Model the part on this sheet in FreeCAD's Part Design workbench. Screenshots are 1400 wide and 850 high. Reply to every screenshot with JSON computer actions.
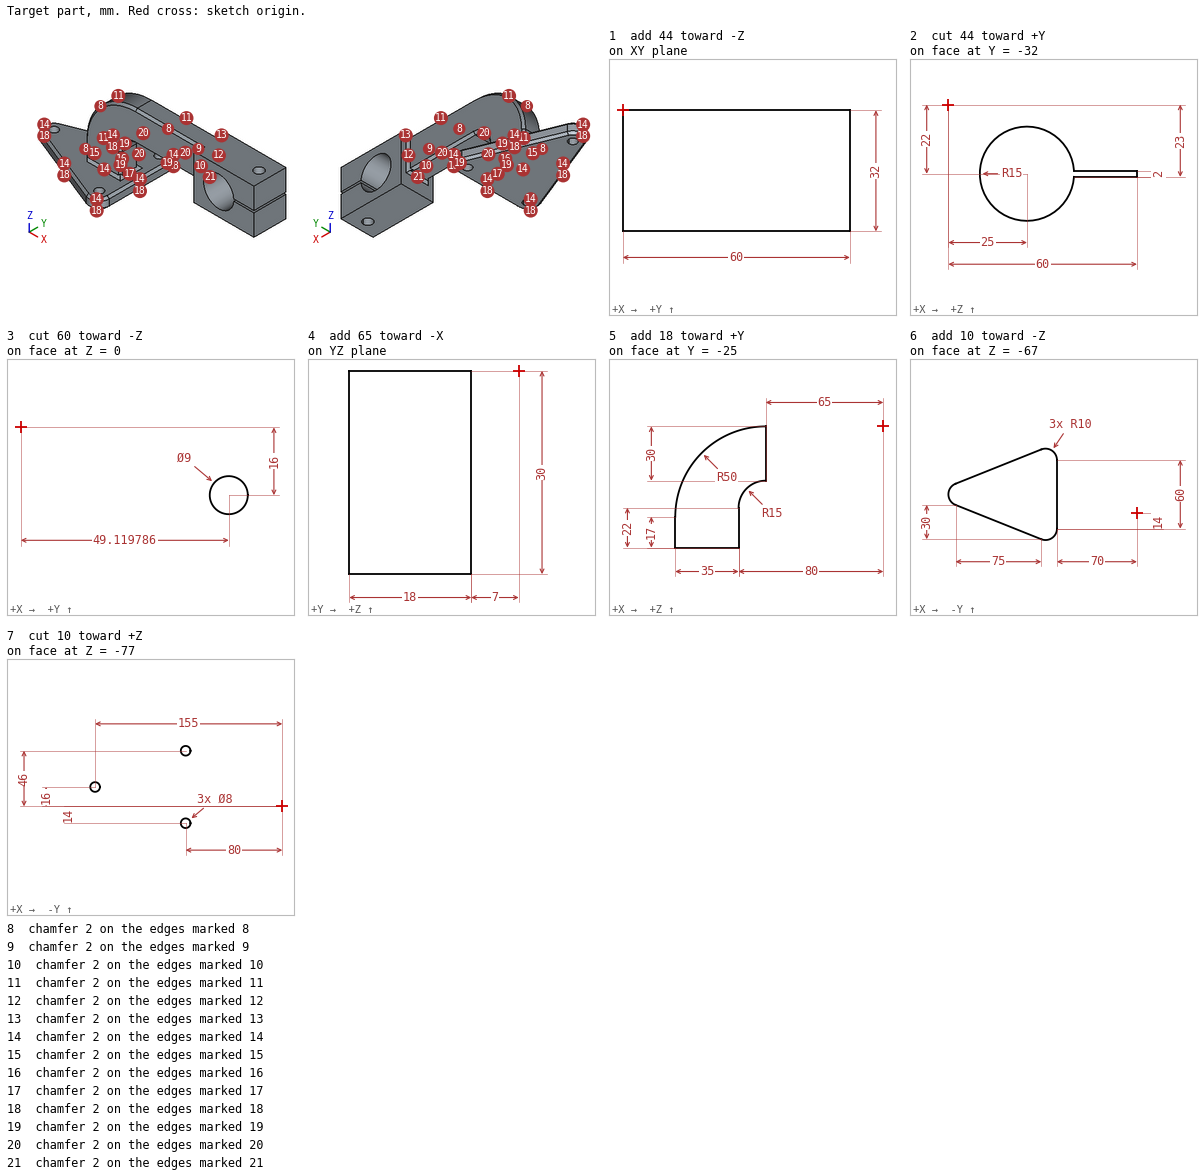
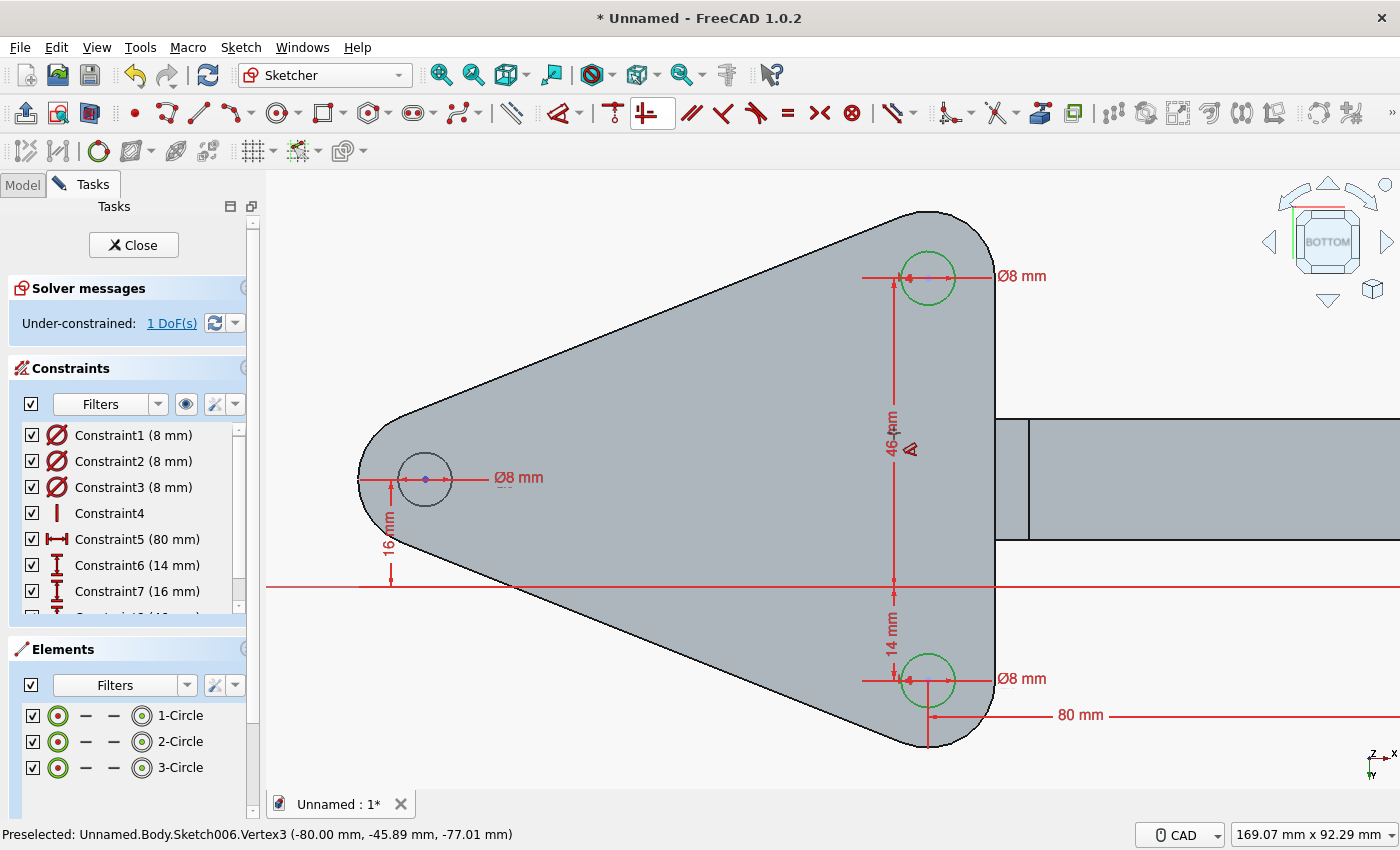
{"action": "left_click", "coordinate": [425, 480]}
{"action": "left_click", "coordinate": [644, 621]}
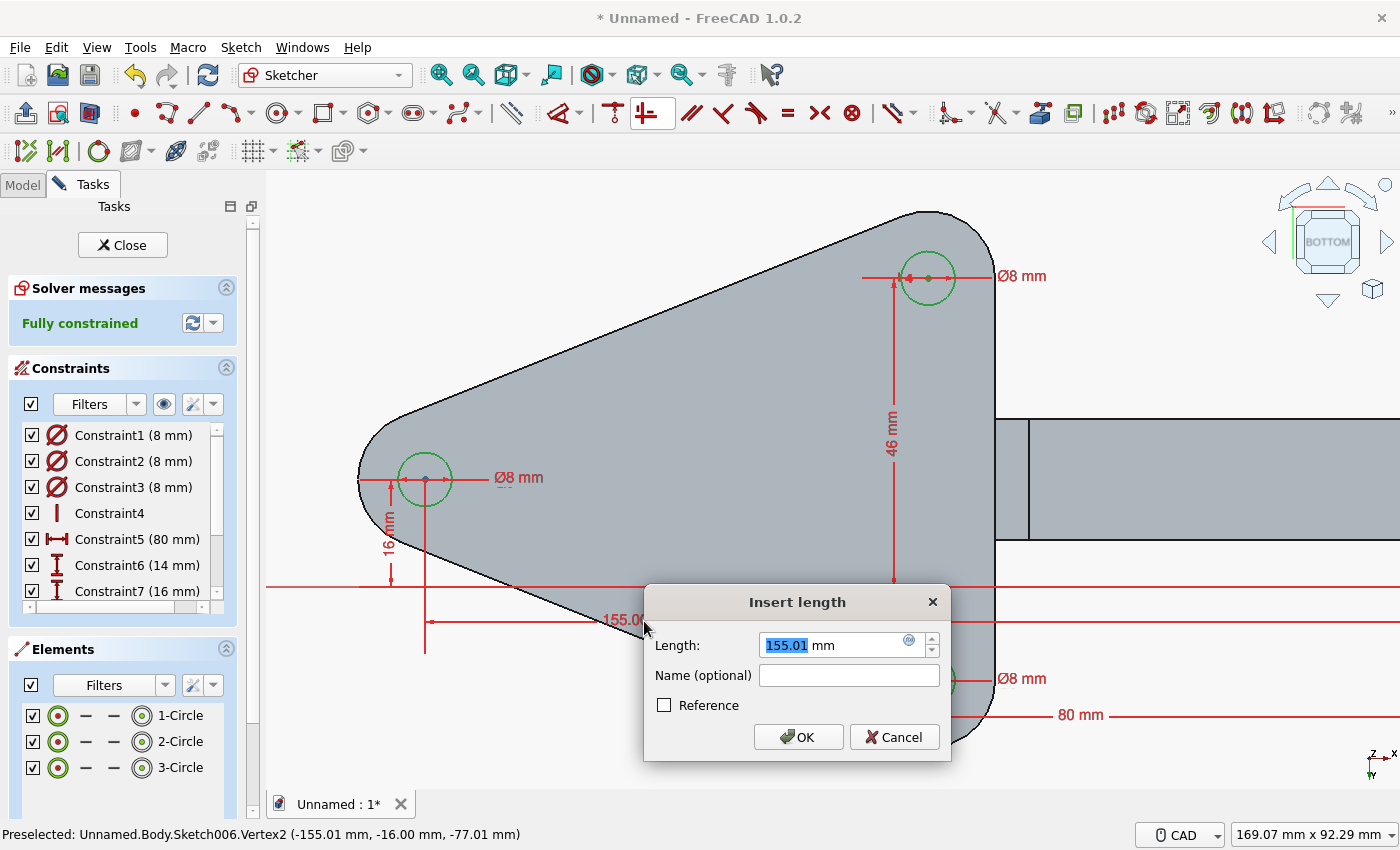
{"action": "type", "text": "155"}
{"action": "key", "text": "Return"}
{"action": "key", "text": "Escape"}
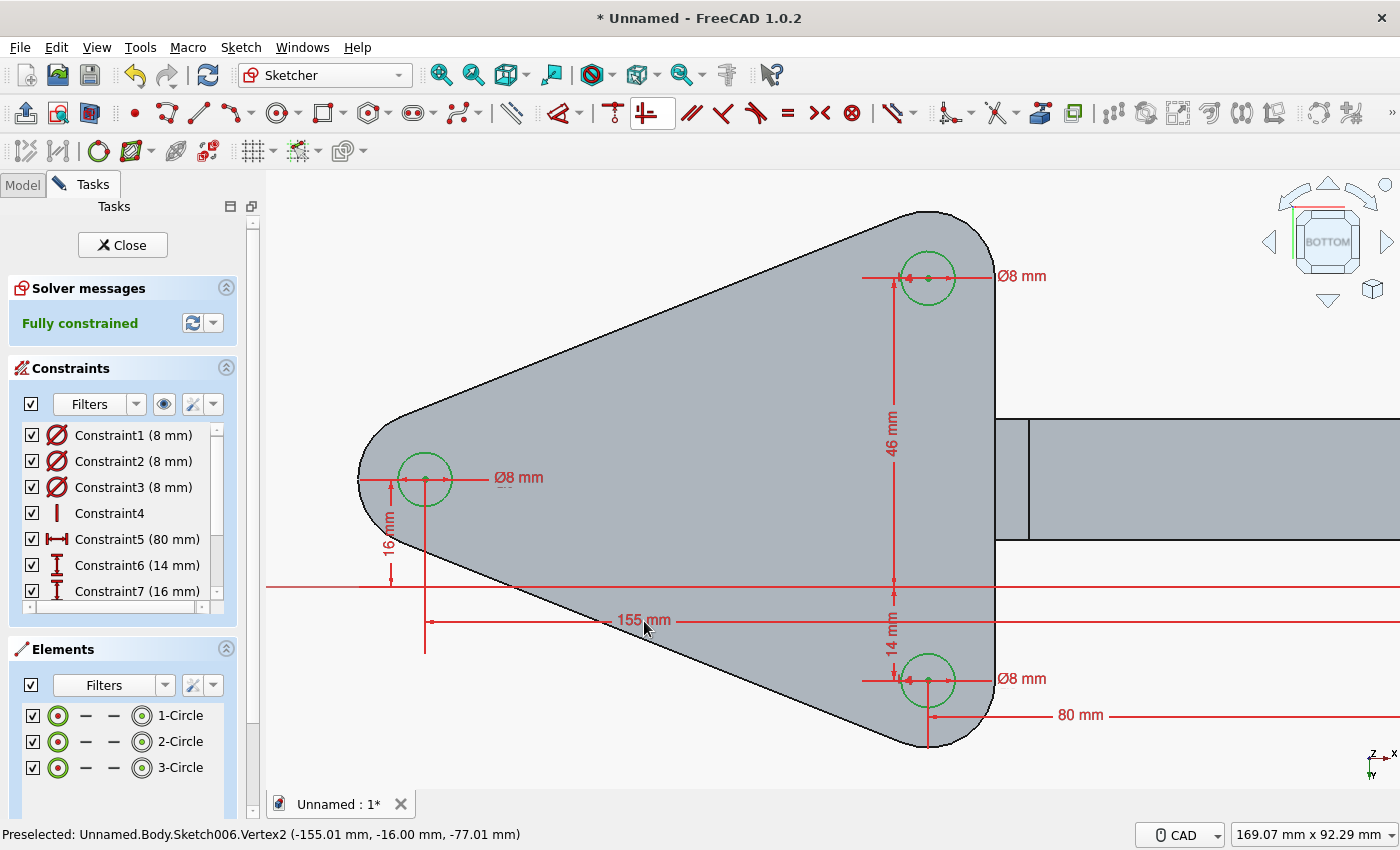
{"action": "left_click", "coordinate": [123, 245]}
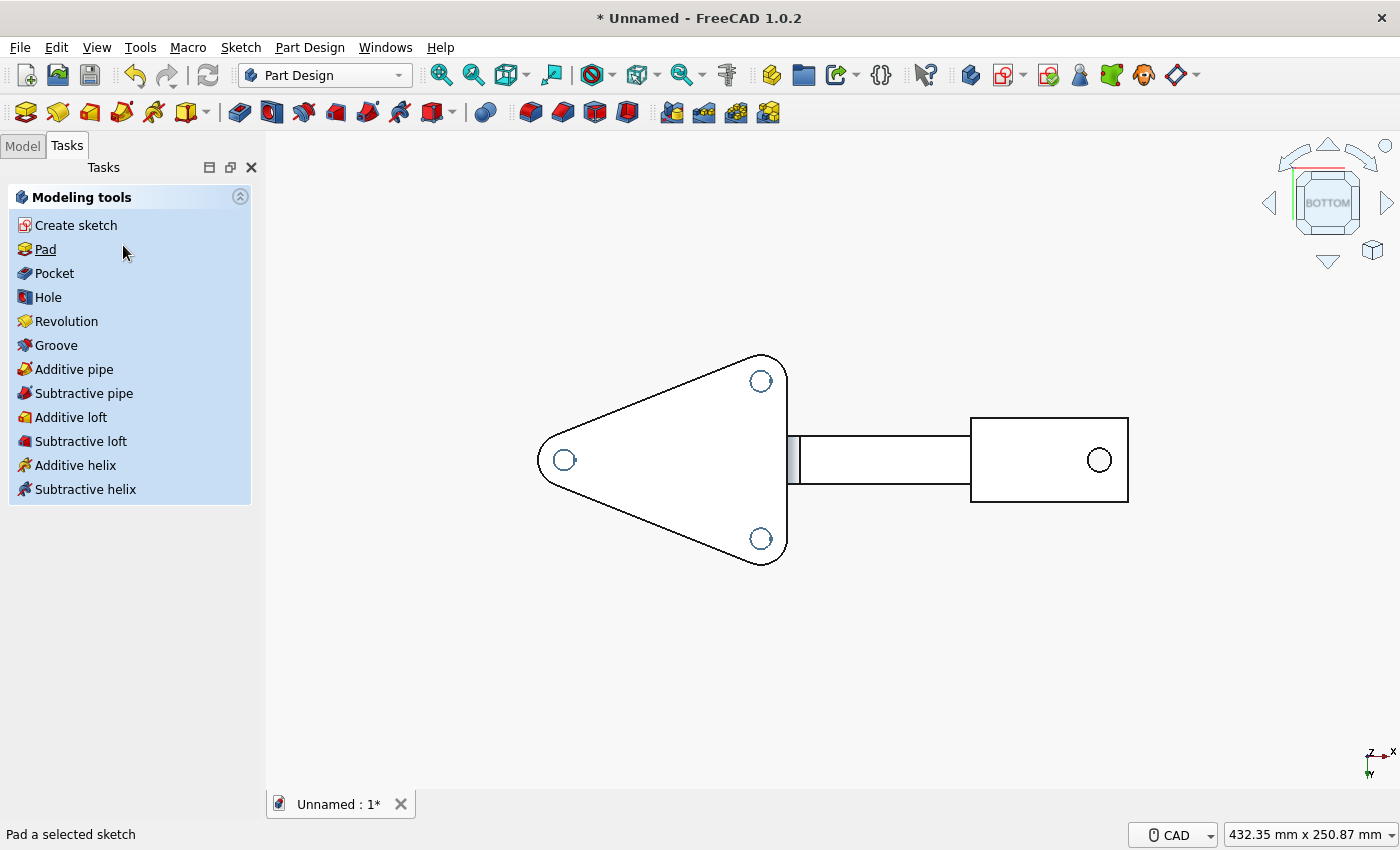
{"action": "left_click", "coordinate": [240, 112]}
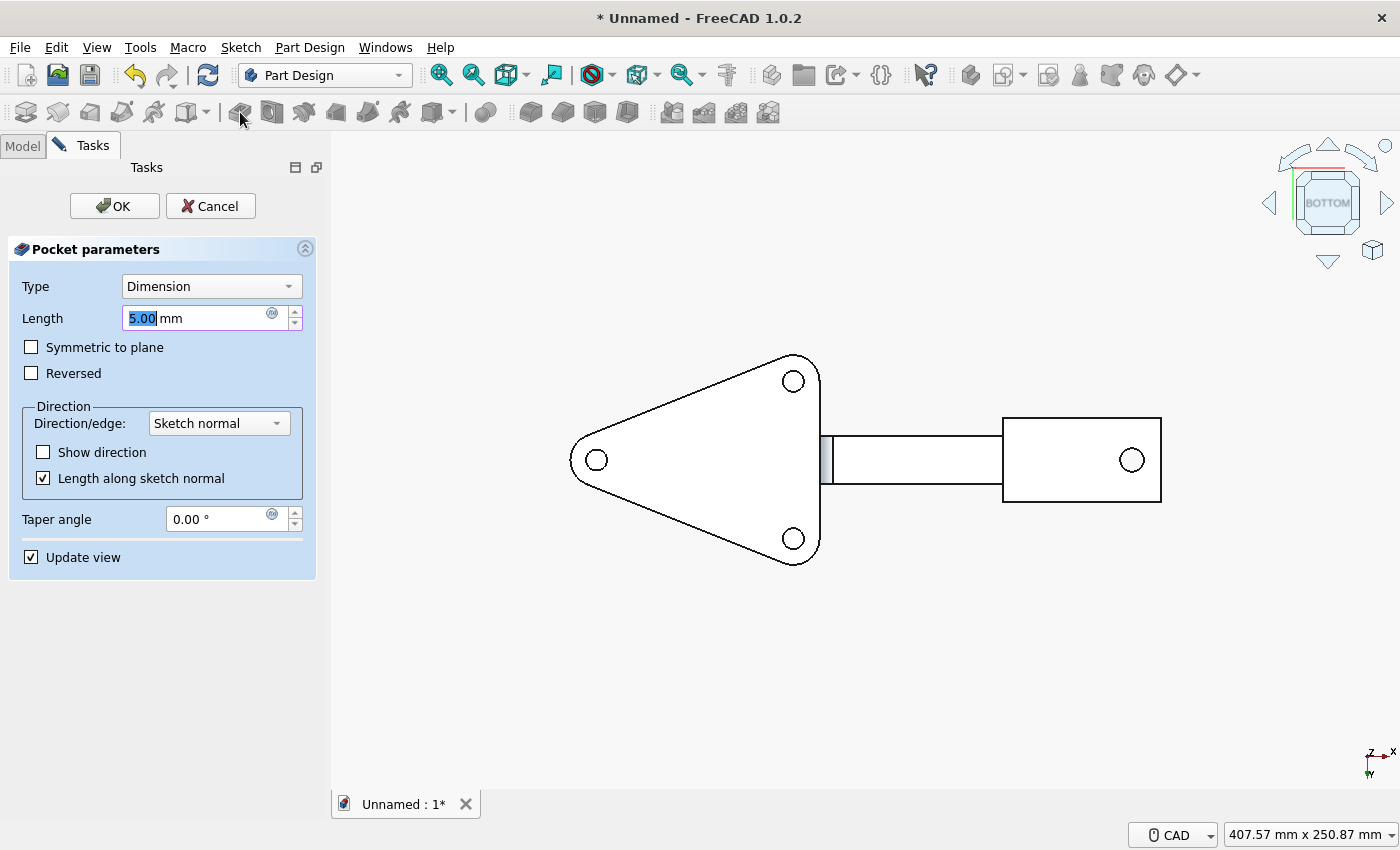
{"action": "type", "text": "10"}
{"action": "key", "text": "Tab"}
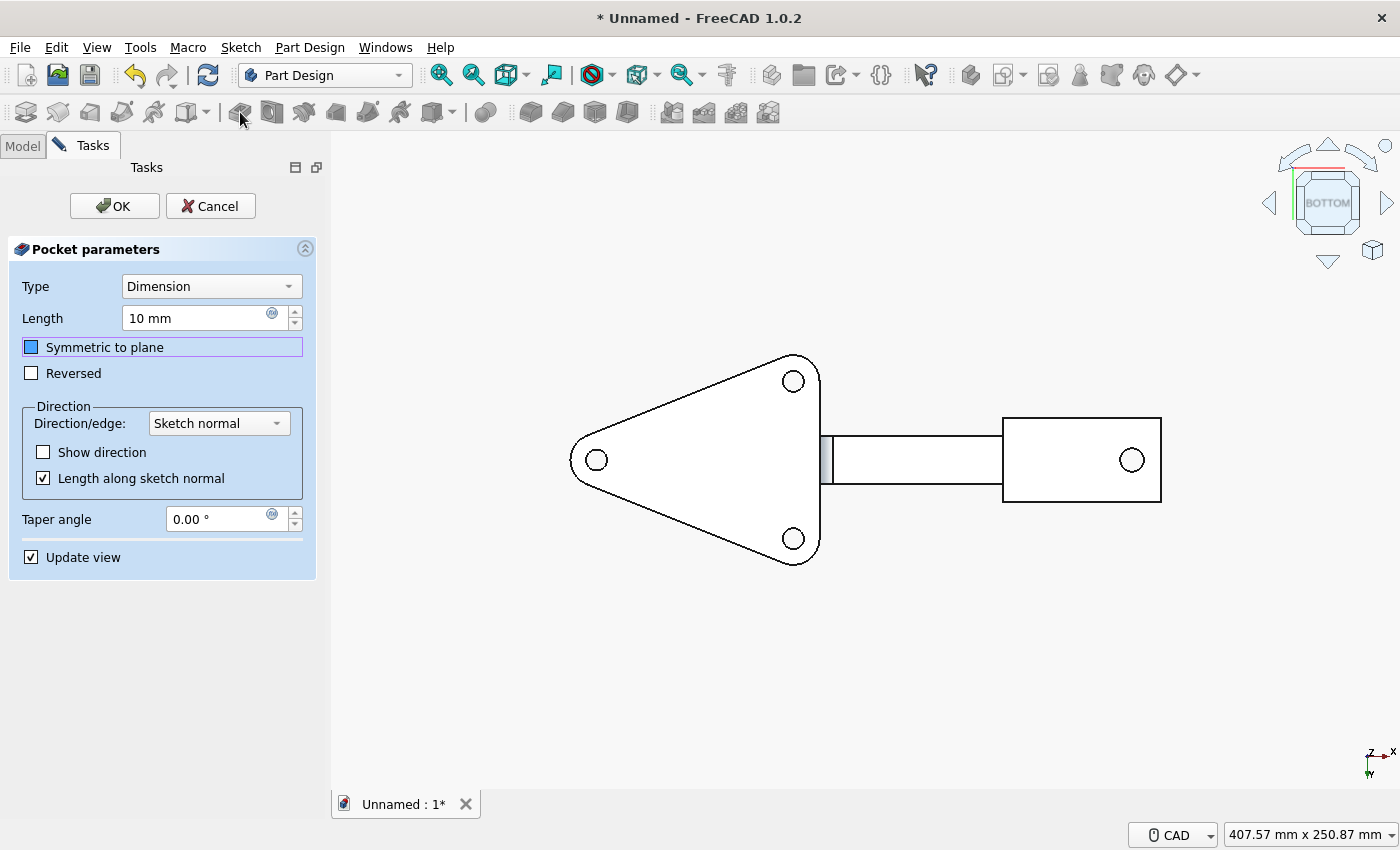
{"action": "left_click", "coordinate": [115, 206]}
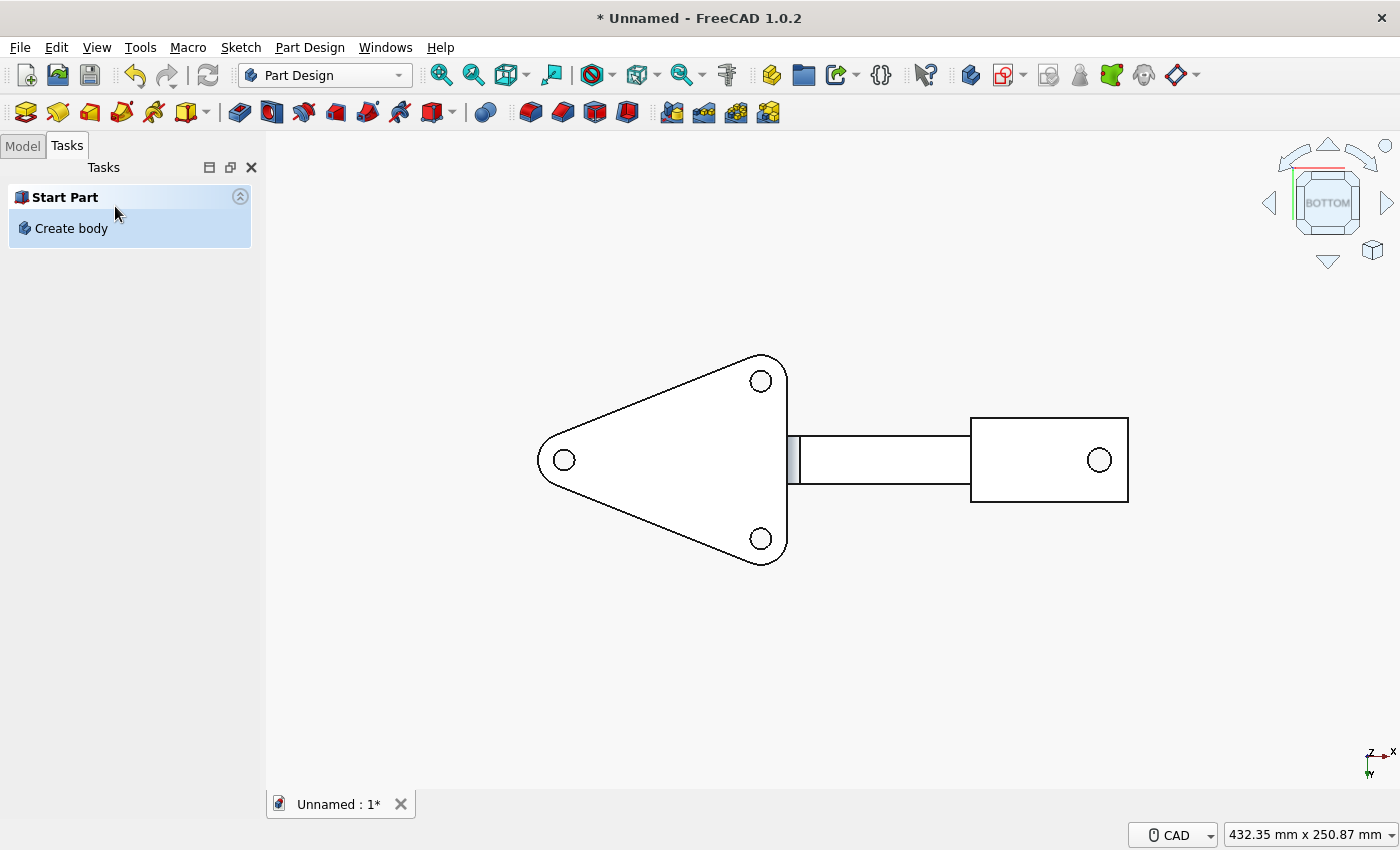
{"action": "key", "text": "0"}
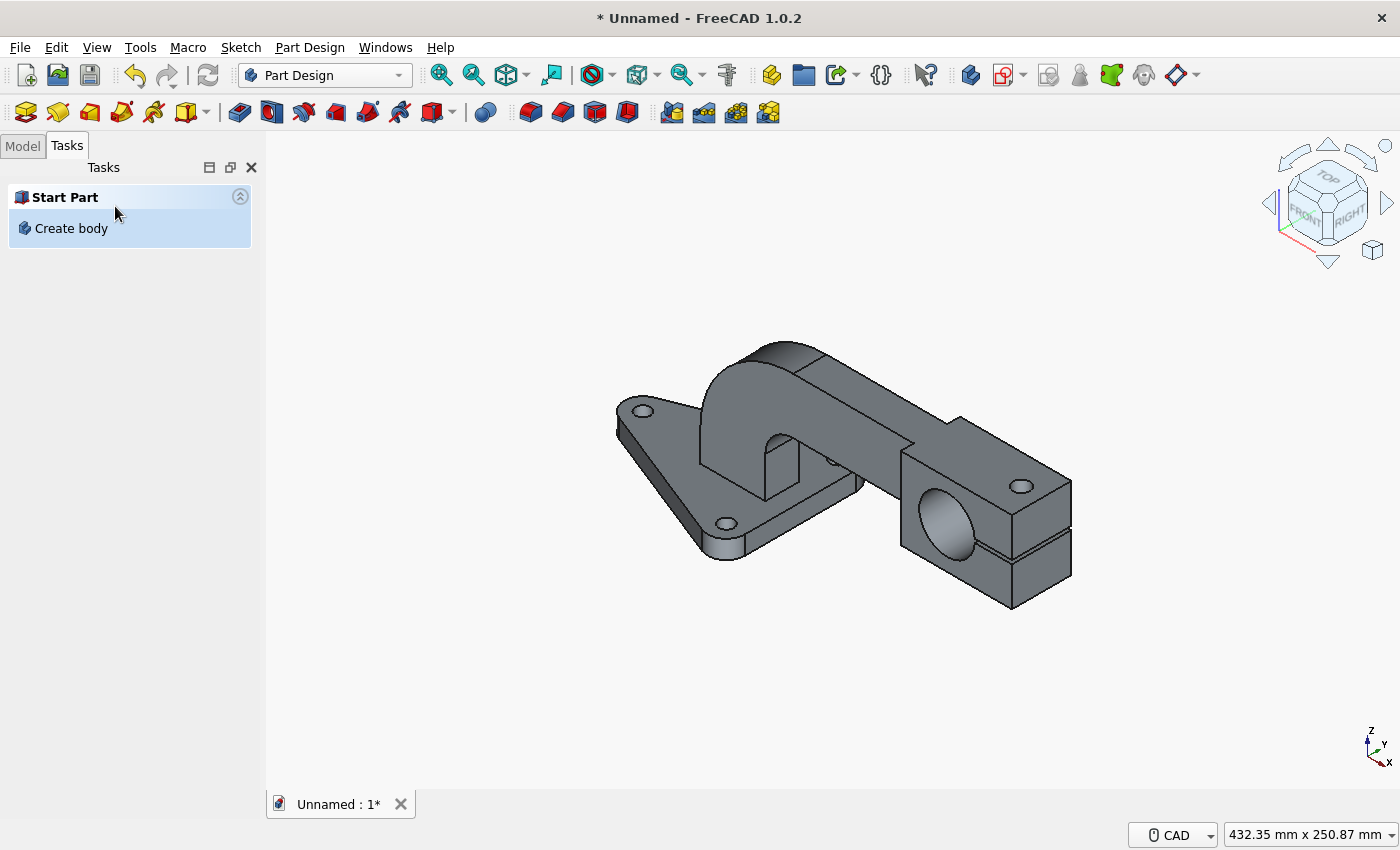
{"action": "left_click", "coordinate": [853, 408]}